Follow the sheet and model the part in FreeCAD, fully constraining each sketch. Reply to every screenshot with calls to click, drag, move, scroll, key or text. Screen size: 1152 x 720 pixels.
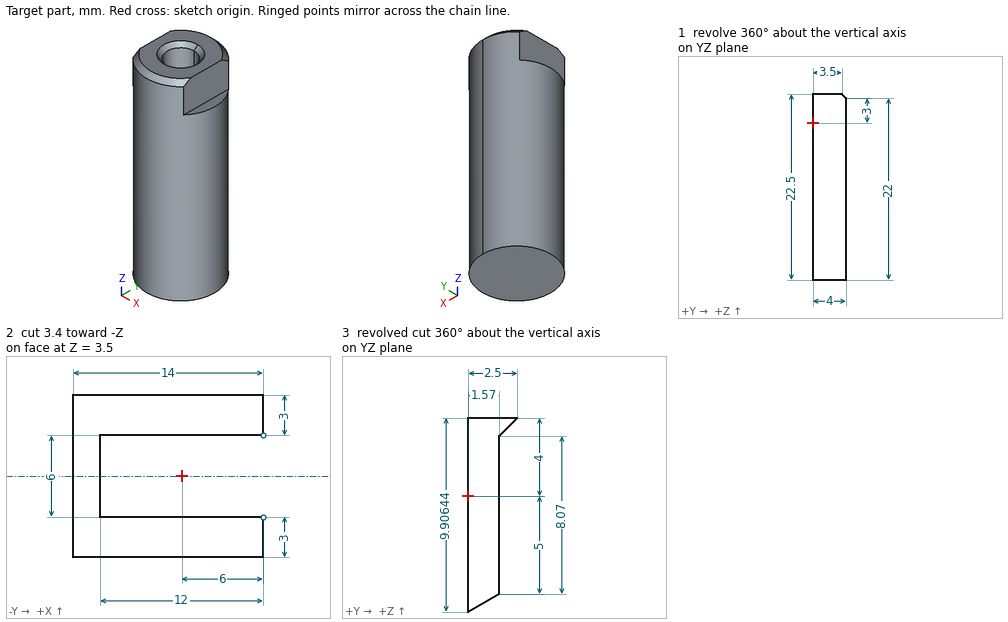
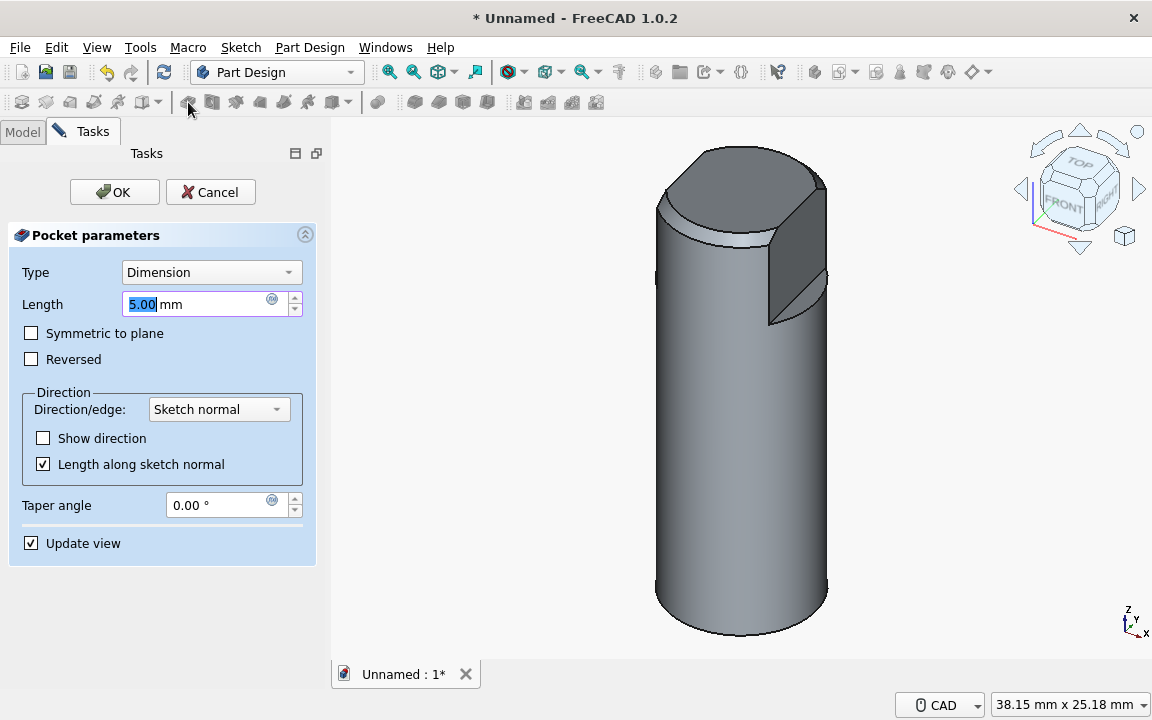
text(3.4)
key(Tab)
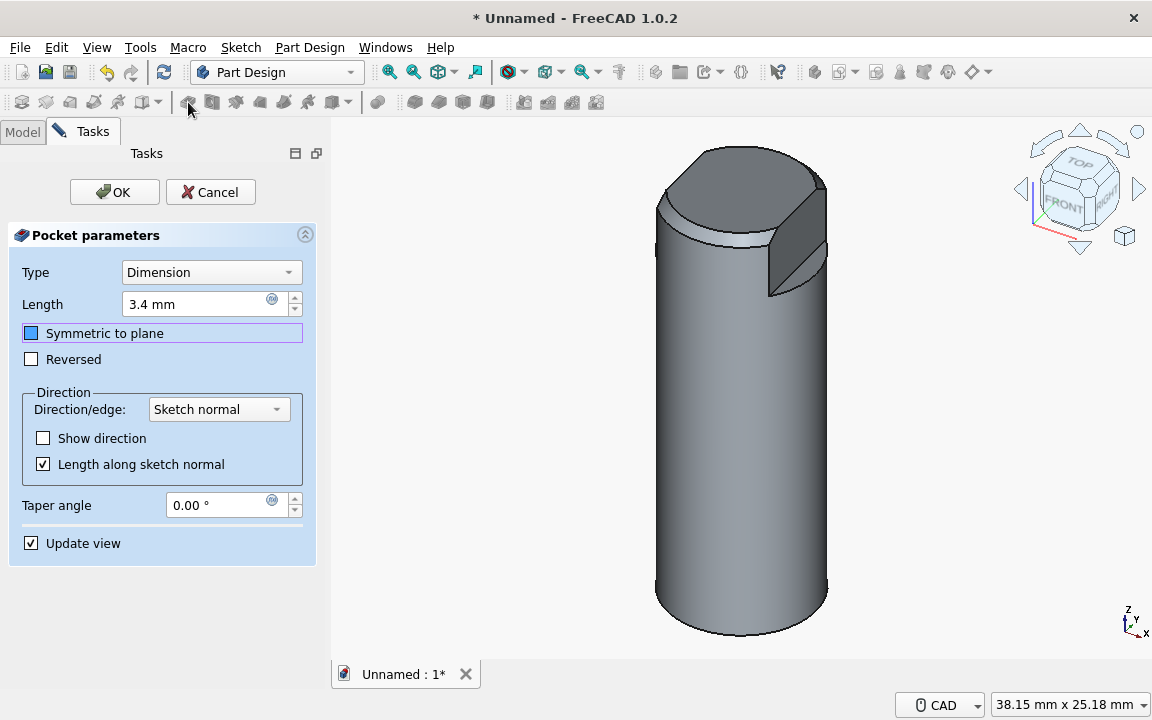
click(115, 192)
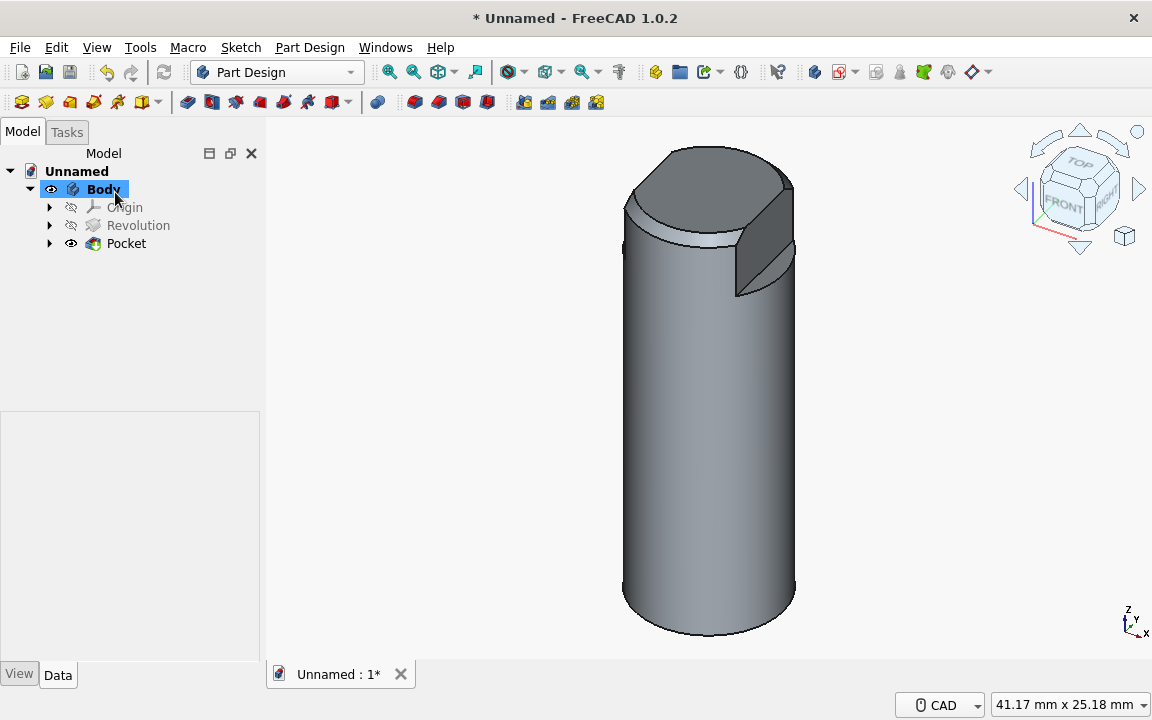
click(840, 72)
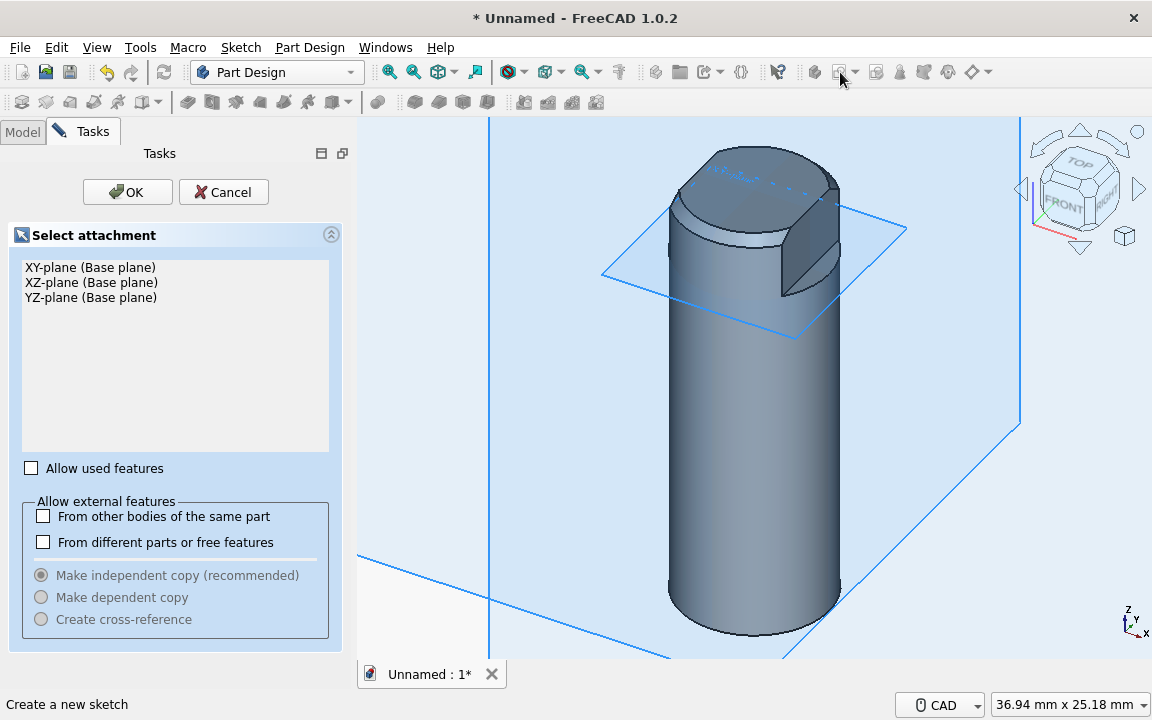
click(82, 298)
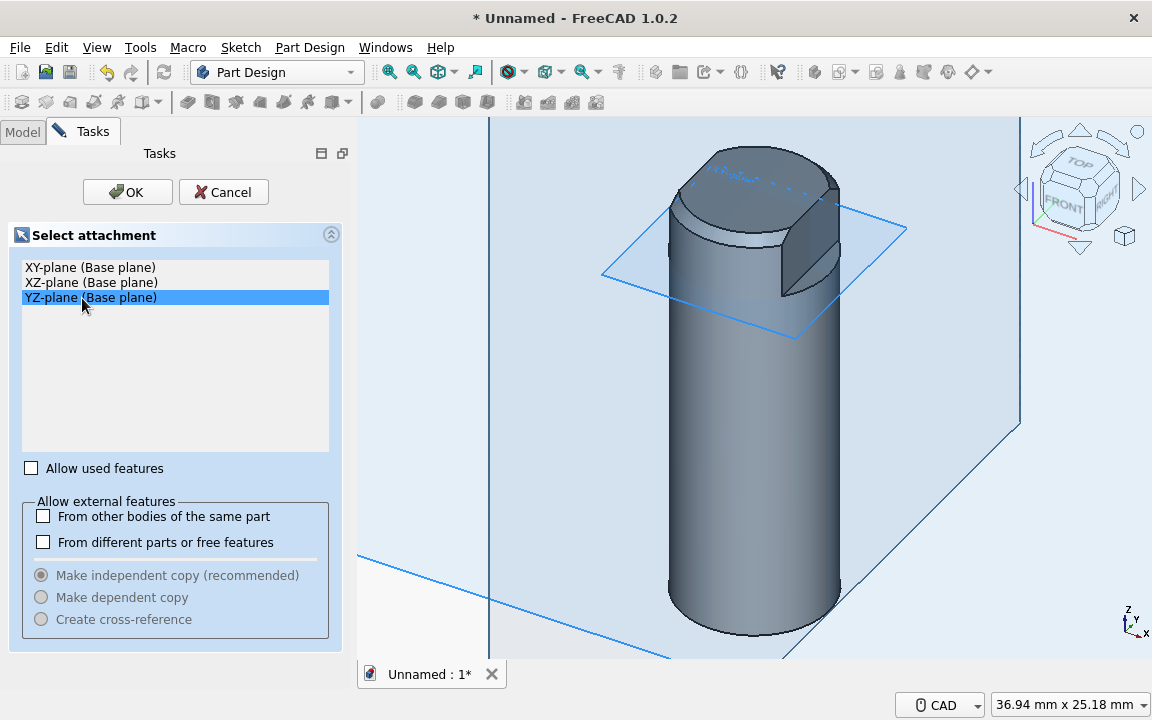
click(128, 192)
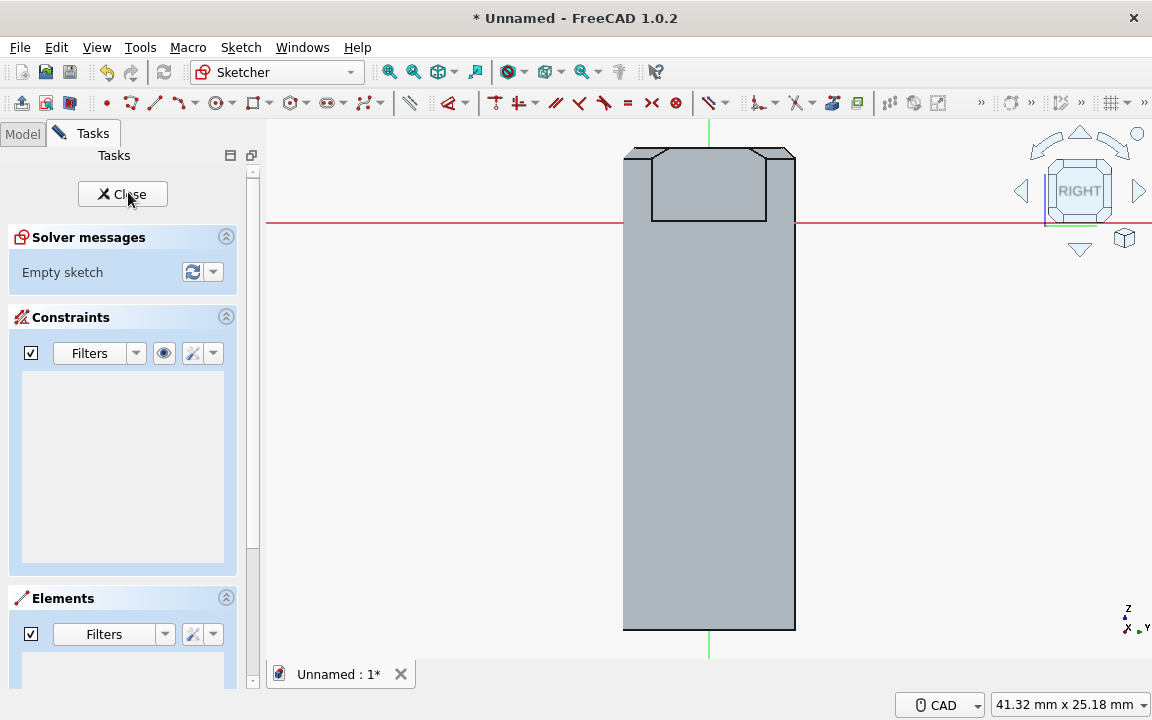
click(70, 104)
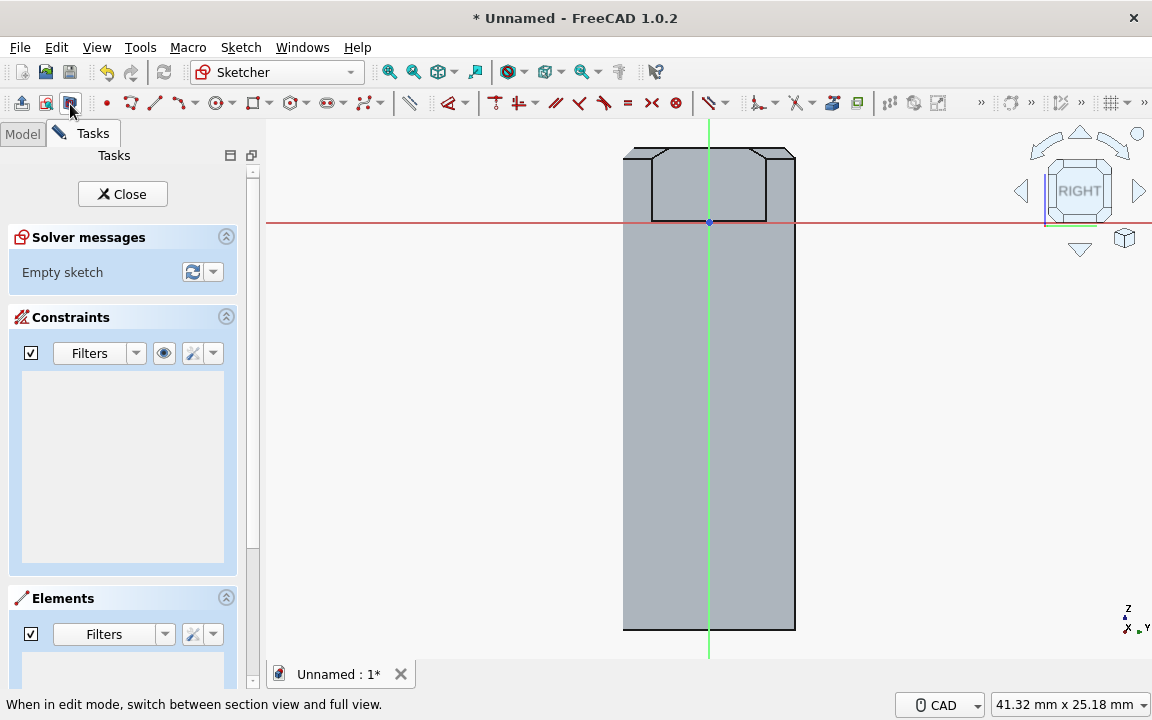
scroll(294, 631, down, 1)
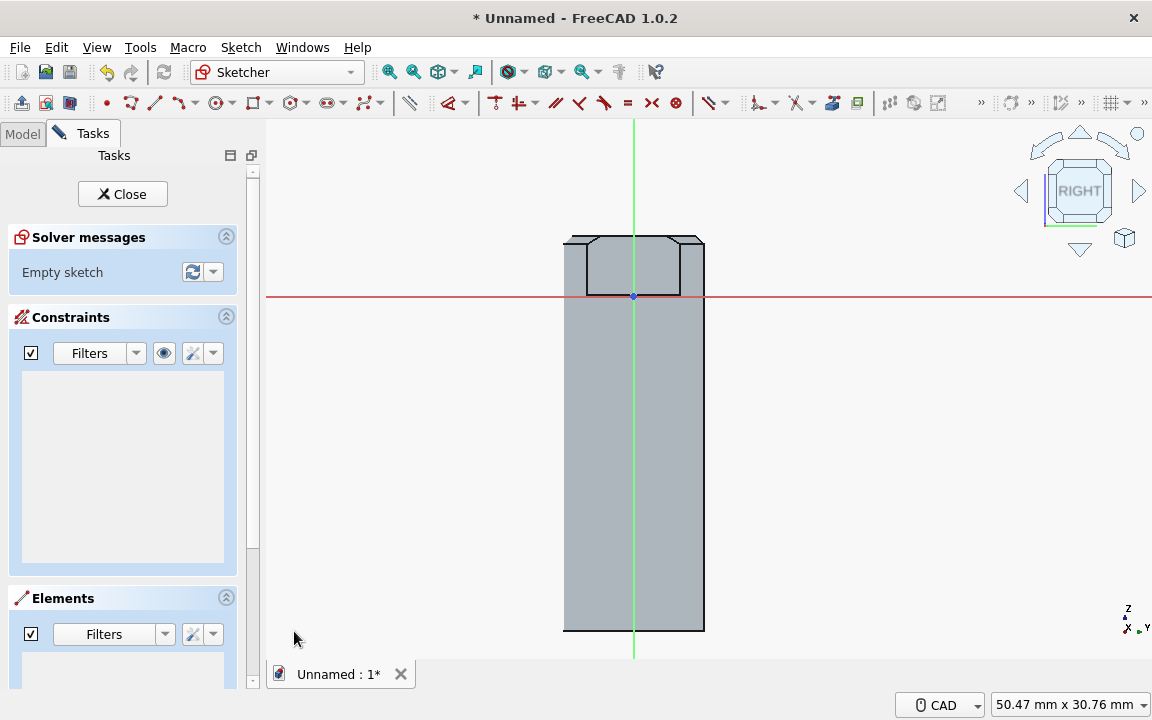
scroll(674, 222, up, 3)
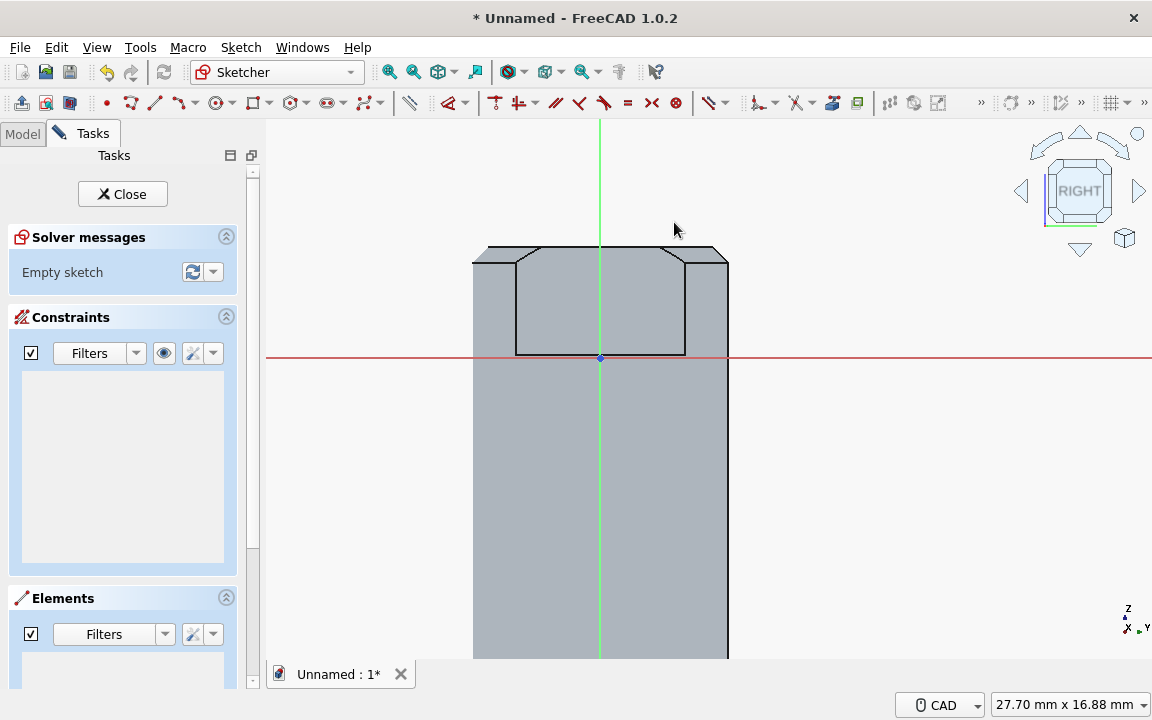
click(132, 104)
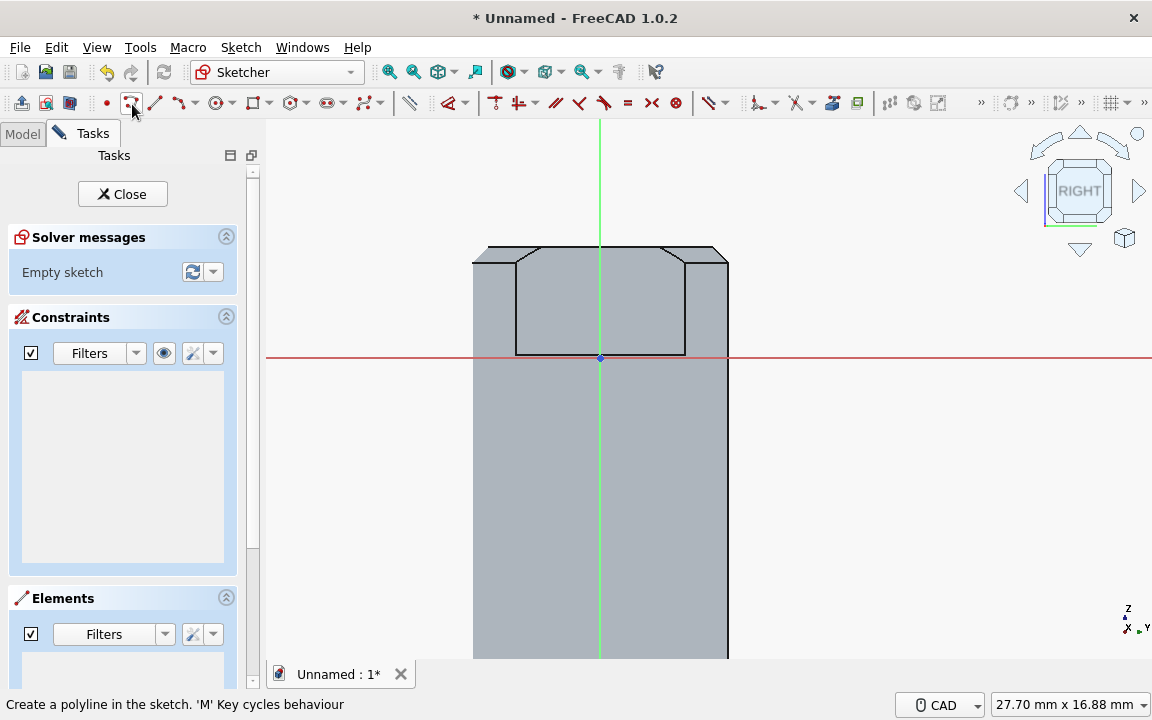
click(651, 260)
click(680, 231)
click(600, 231)
click(609, 547)
click(651, 518)
click(651, 261)
key(Escape)
key(Escape)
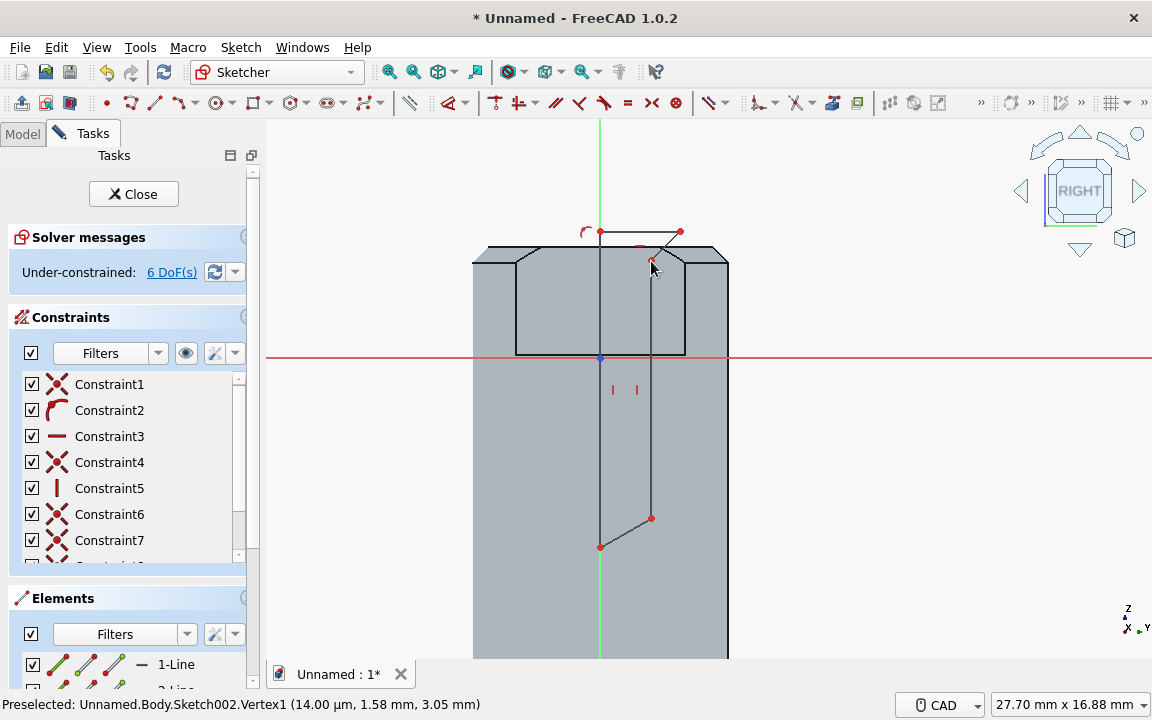
click(448, 104)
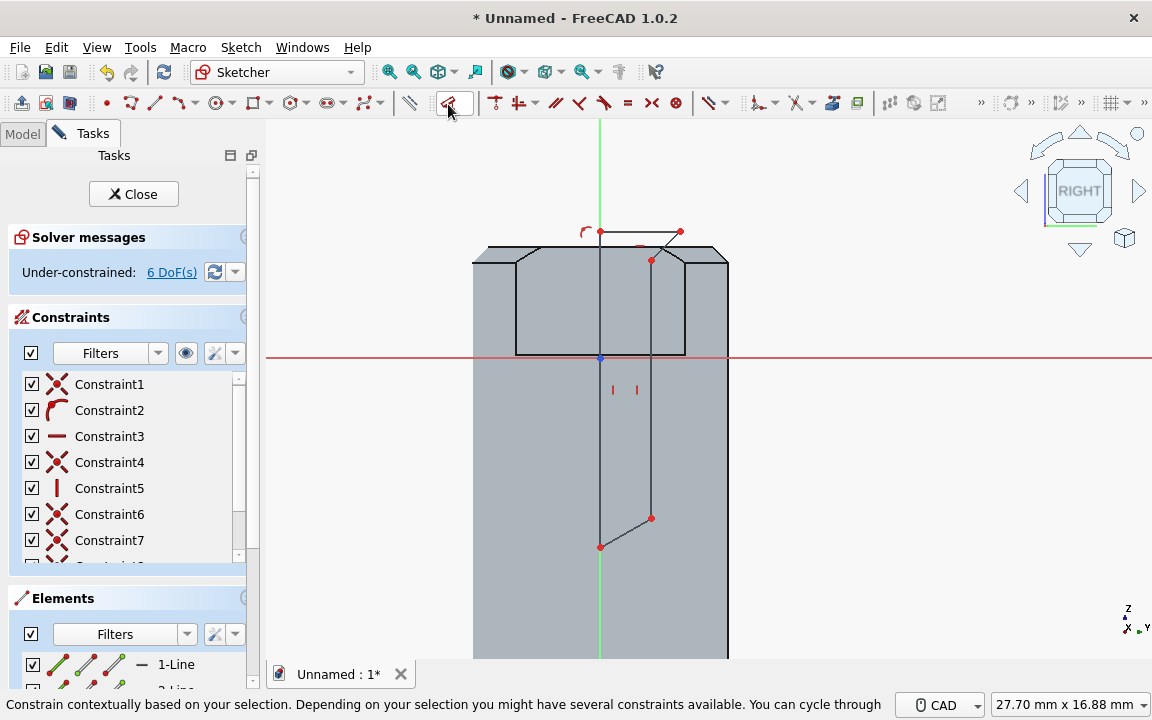
click(680, 232)
click(566, 295)